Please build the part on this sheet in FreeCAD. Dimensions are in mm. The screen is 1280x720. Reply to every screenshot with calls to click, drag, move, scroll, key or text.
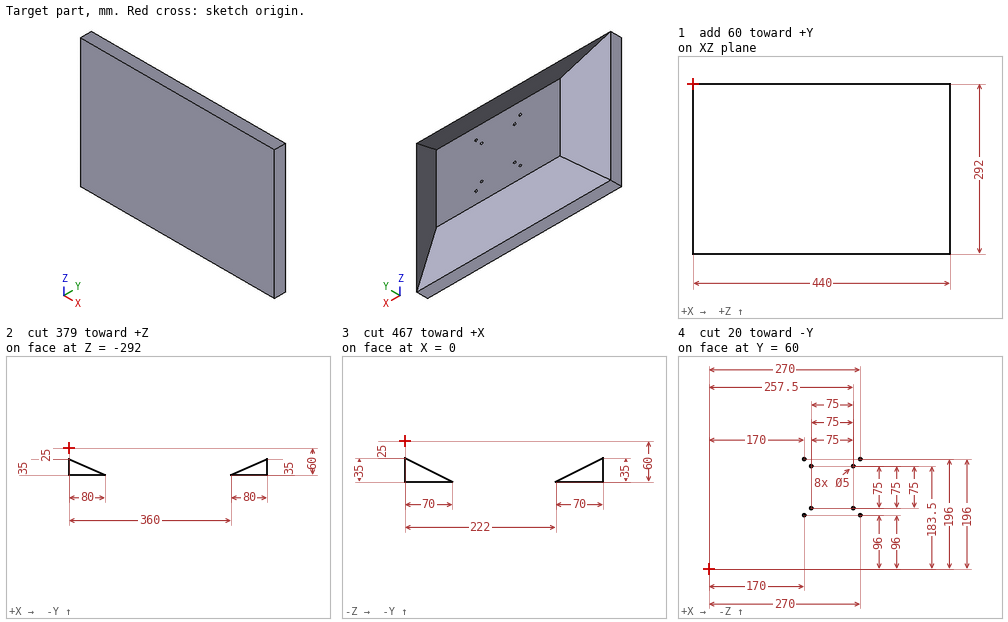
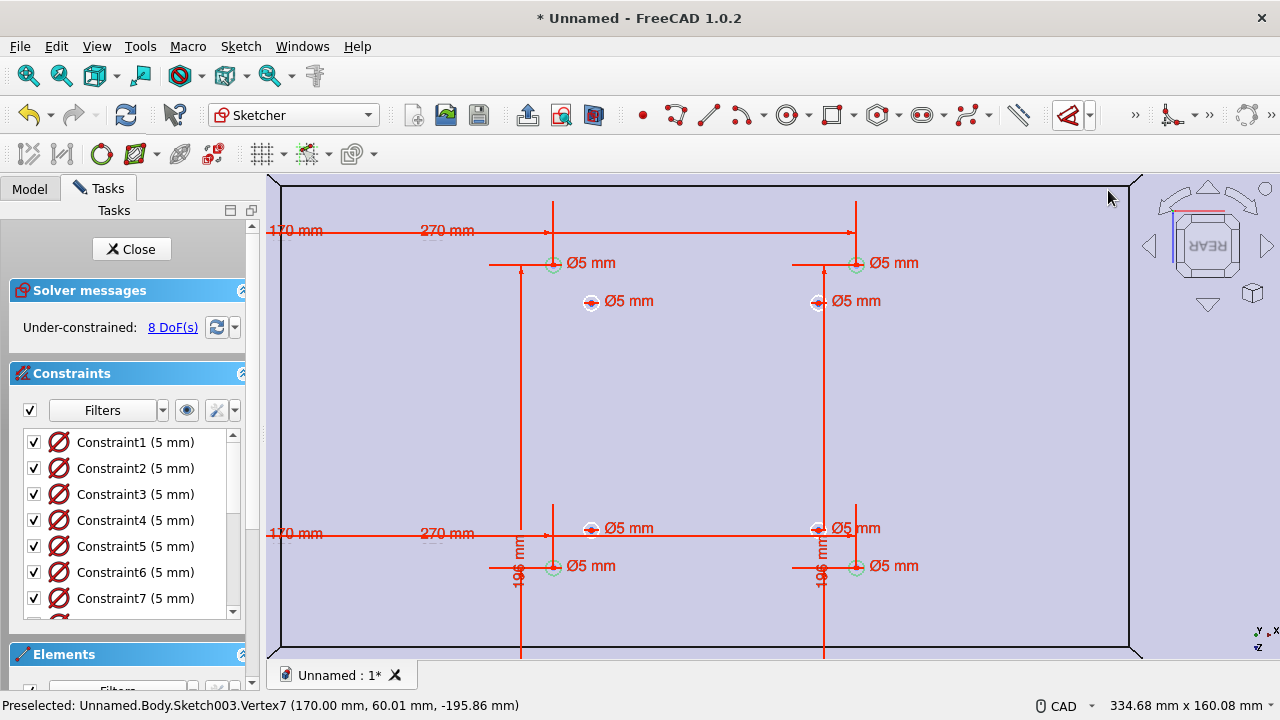
click(819, 303)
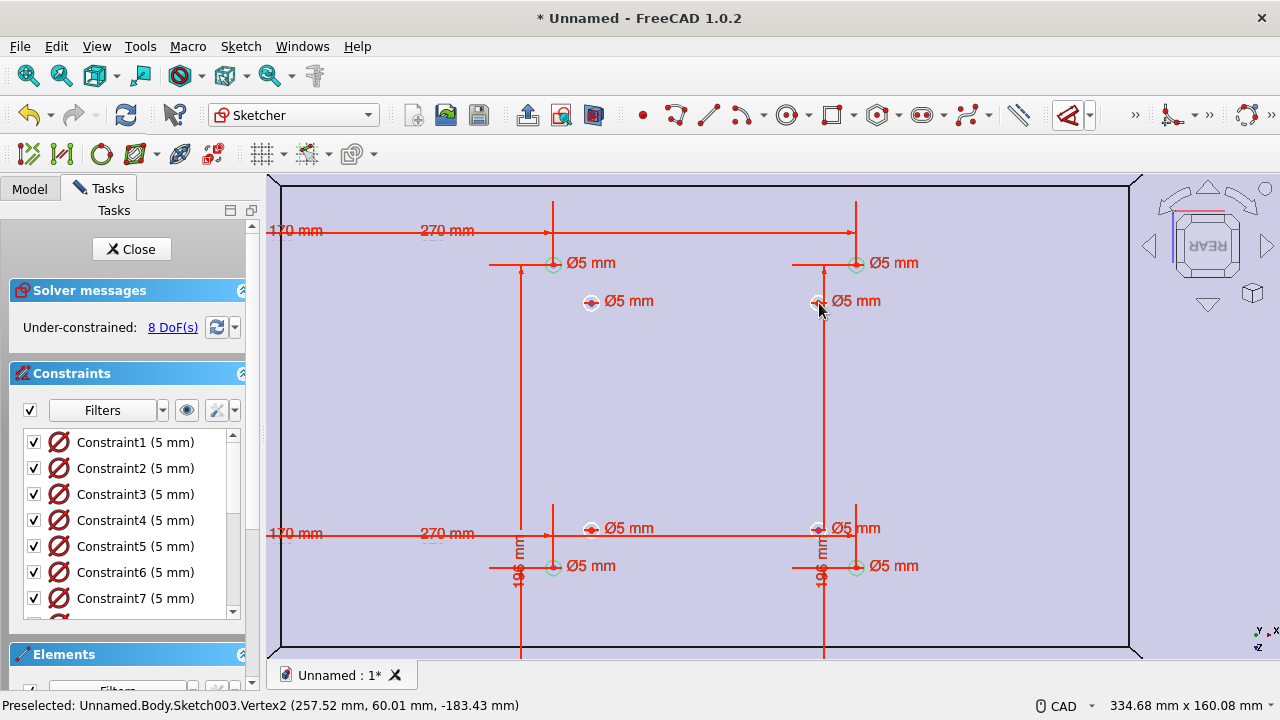
click(818, 530)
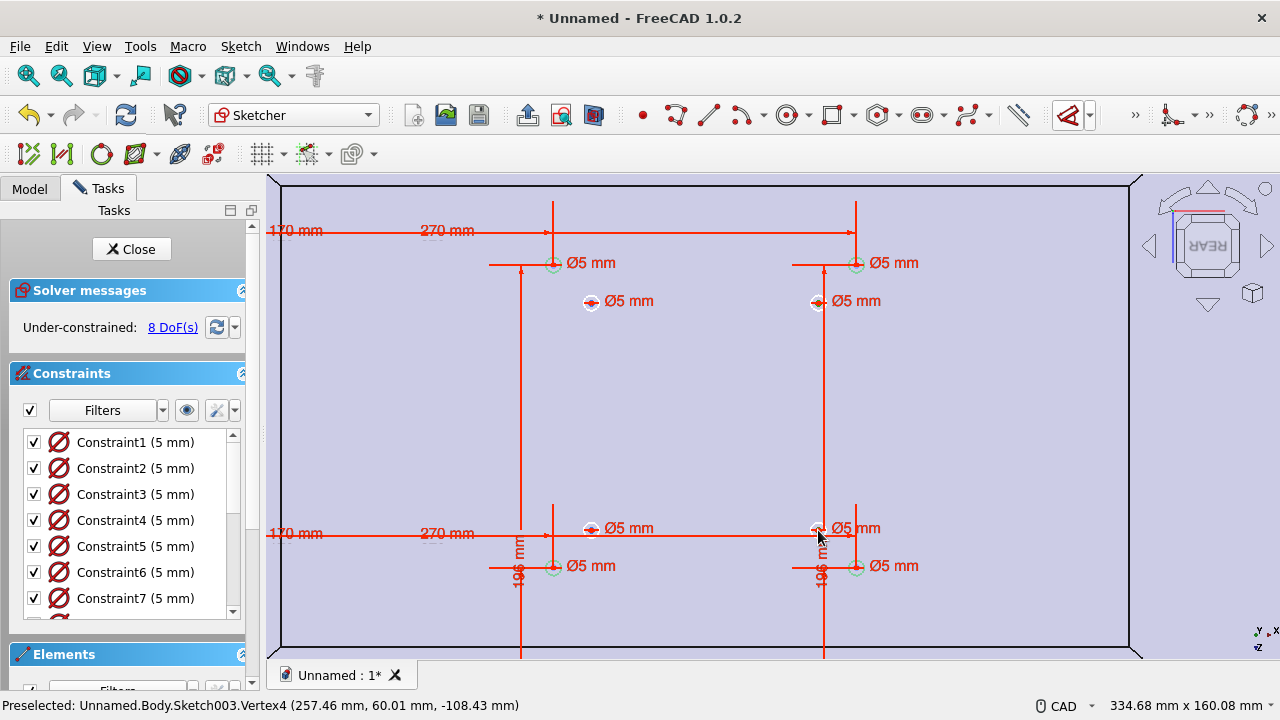
key(i)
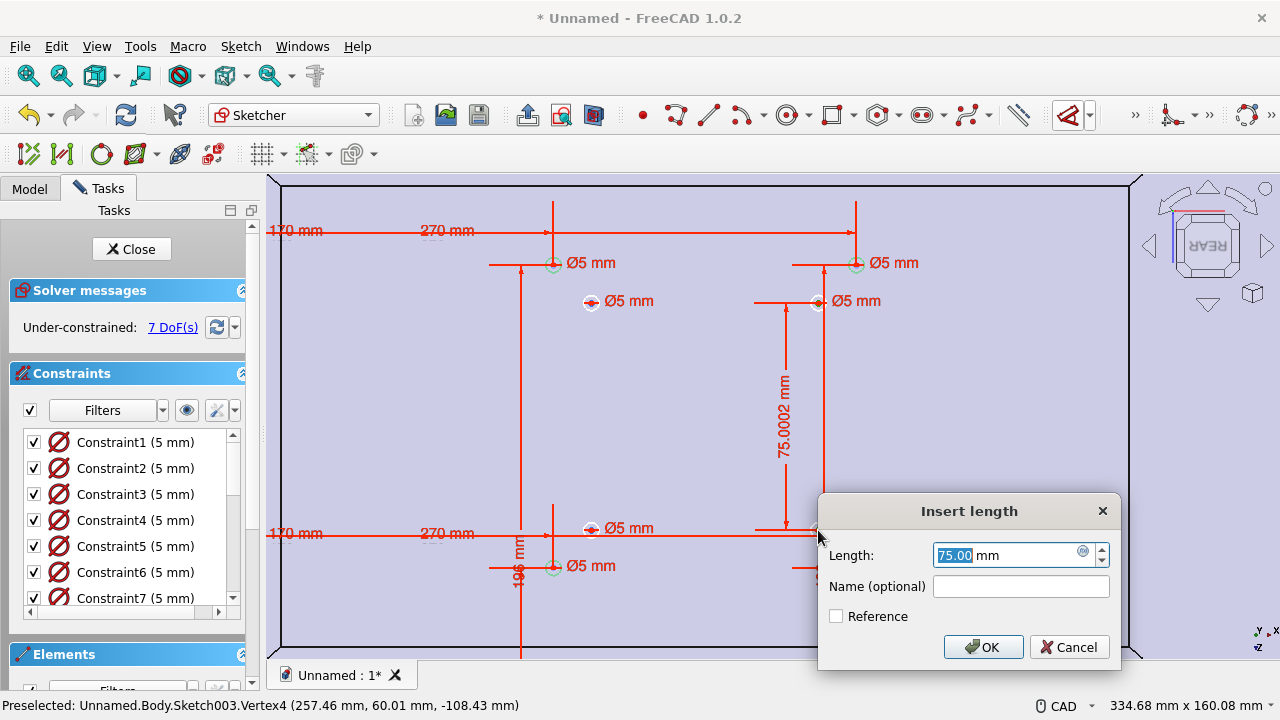
text(75)
key(Return)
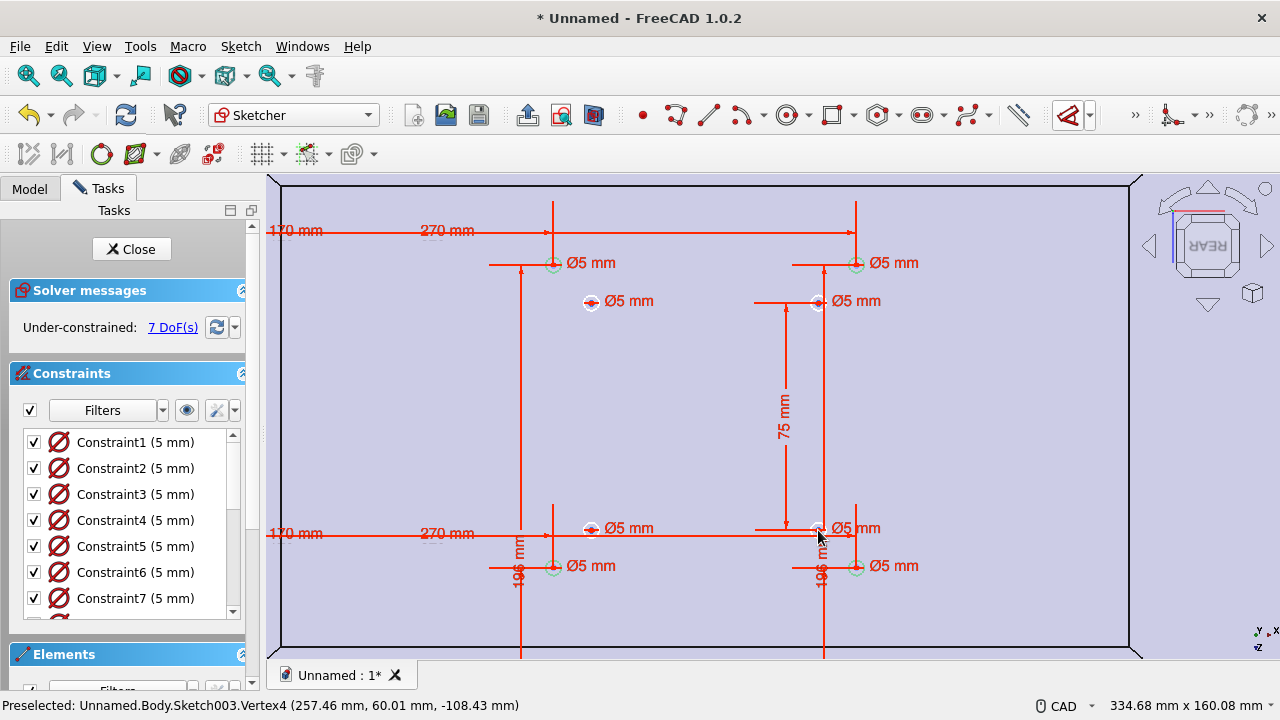
click(818, 530)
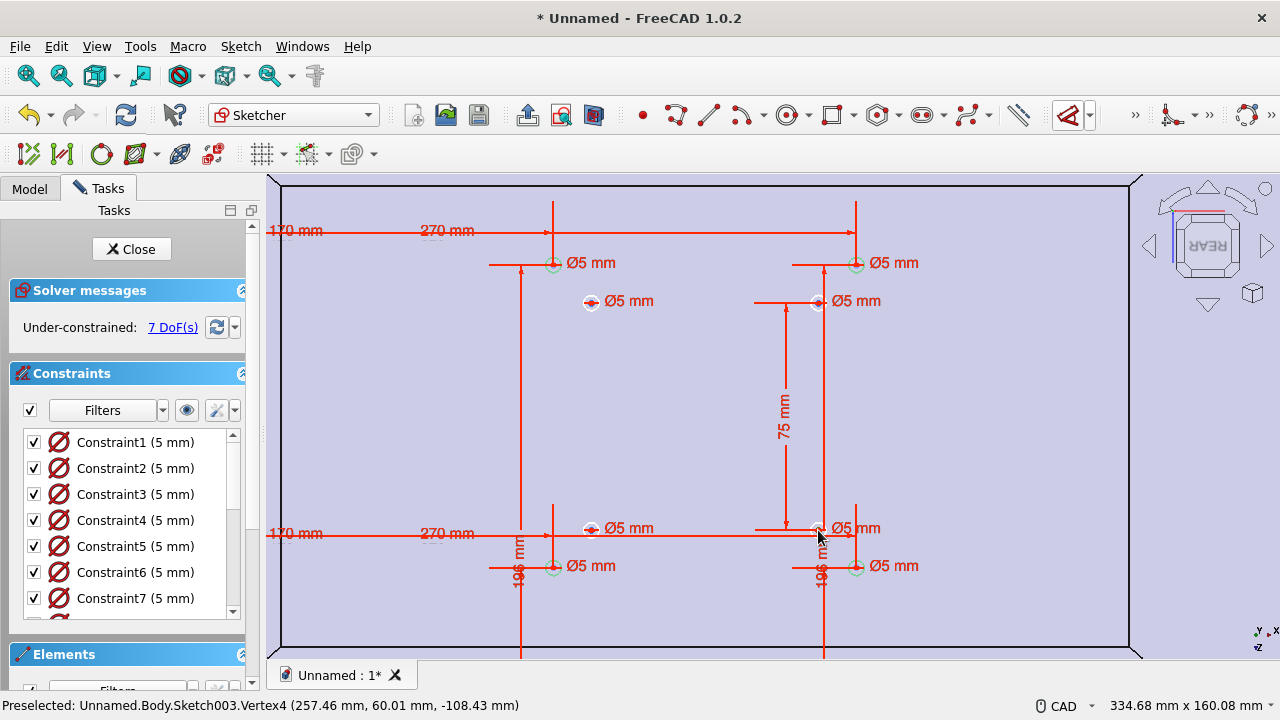
click(591, 530)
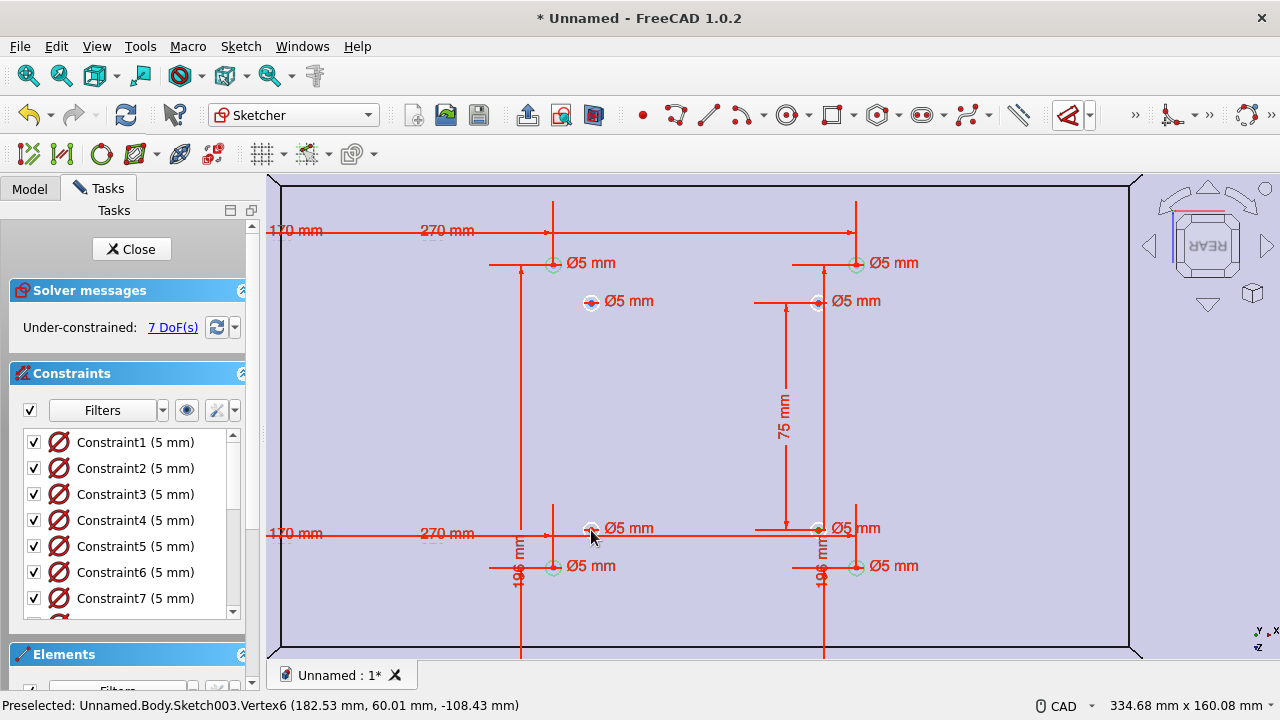
key(l)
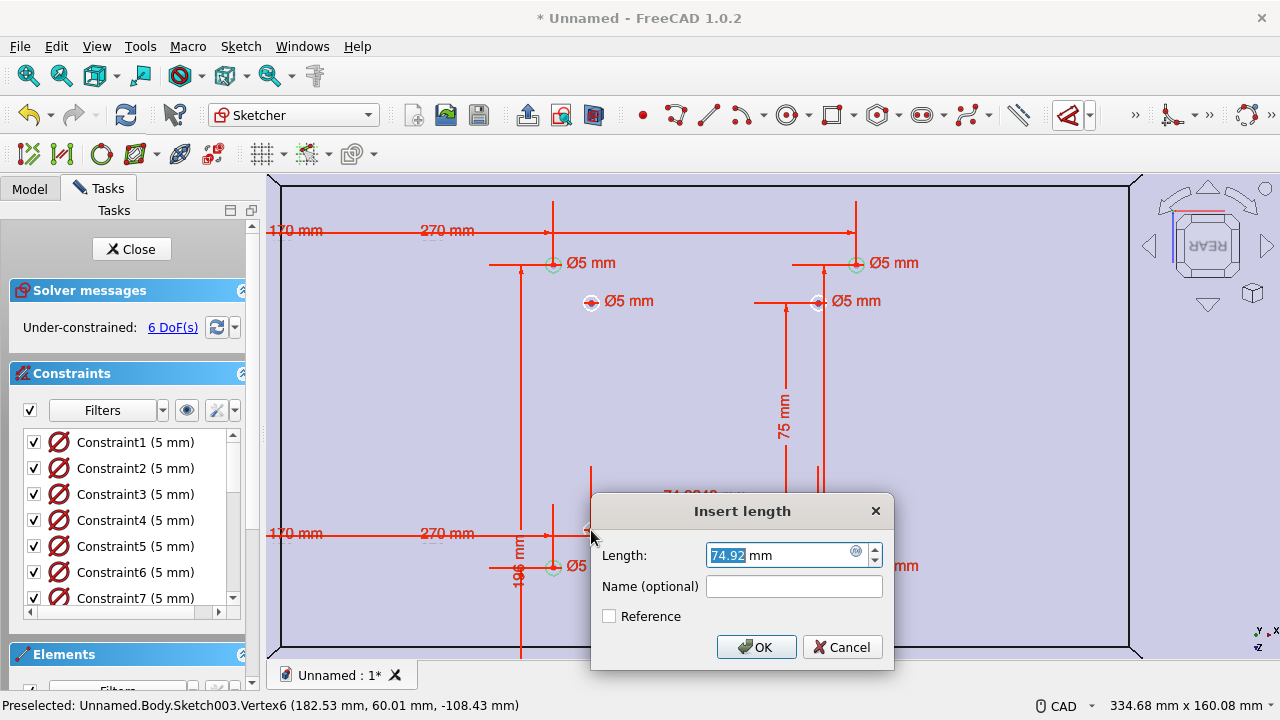
text(75)
key(Return)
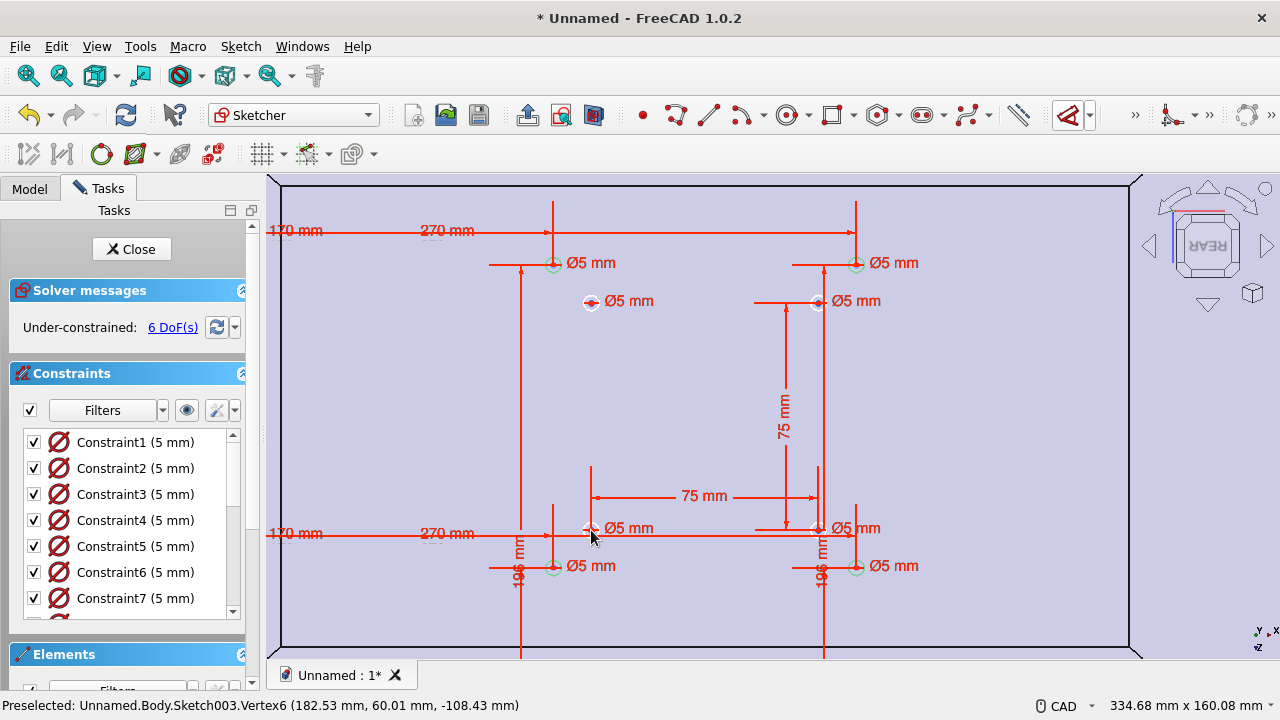
click(819, 303)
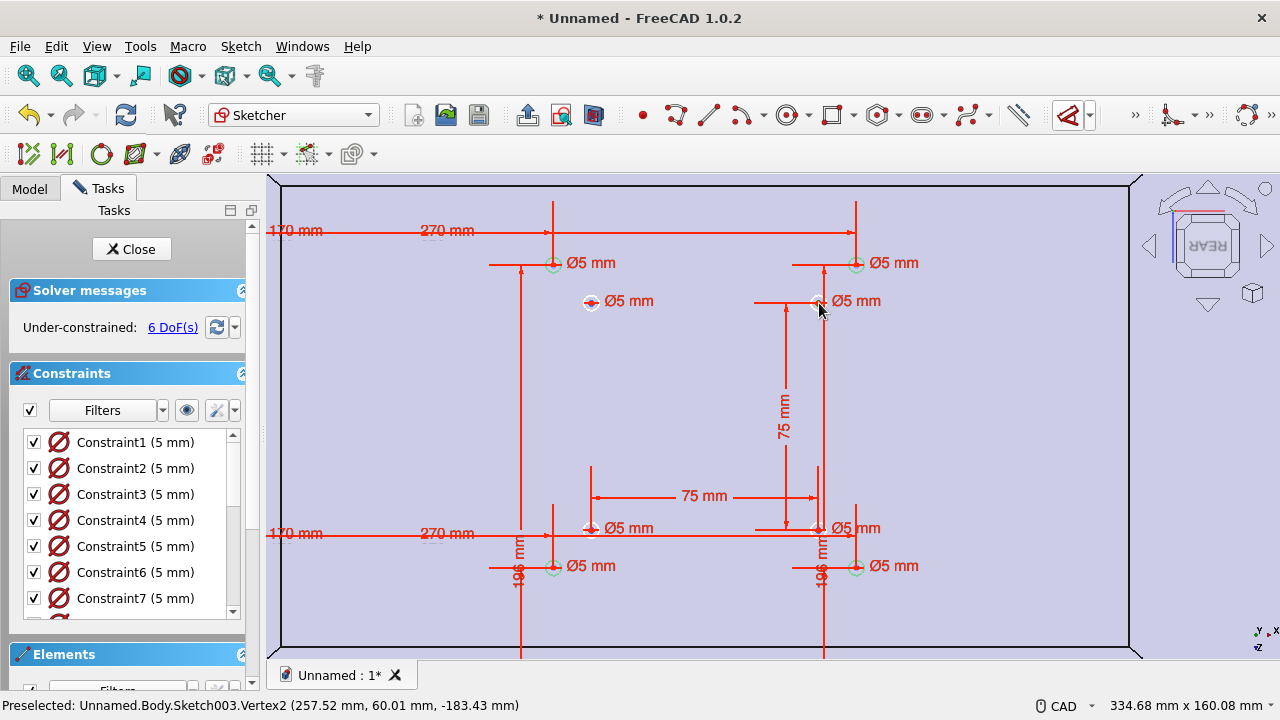
click(591, 530)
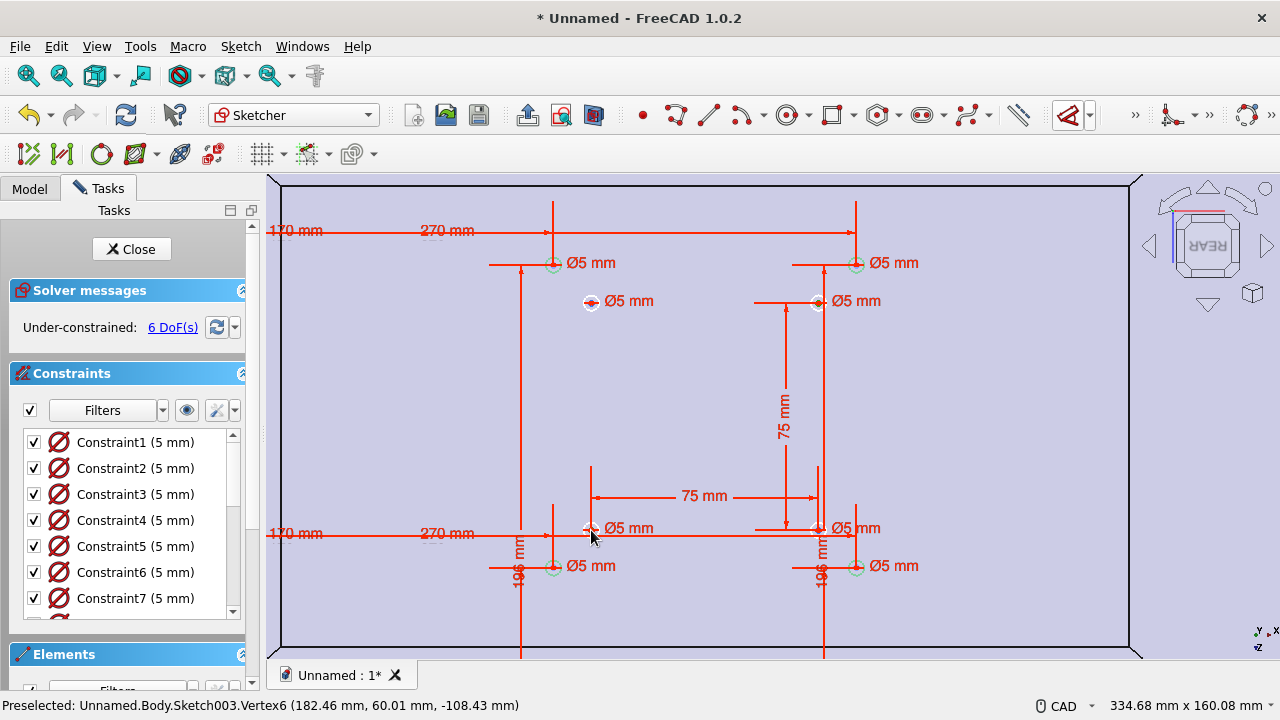
key(l)